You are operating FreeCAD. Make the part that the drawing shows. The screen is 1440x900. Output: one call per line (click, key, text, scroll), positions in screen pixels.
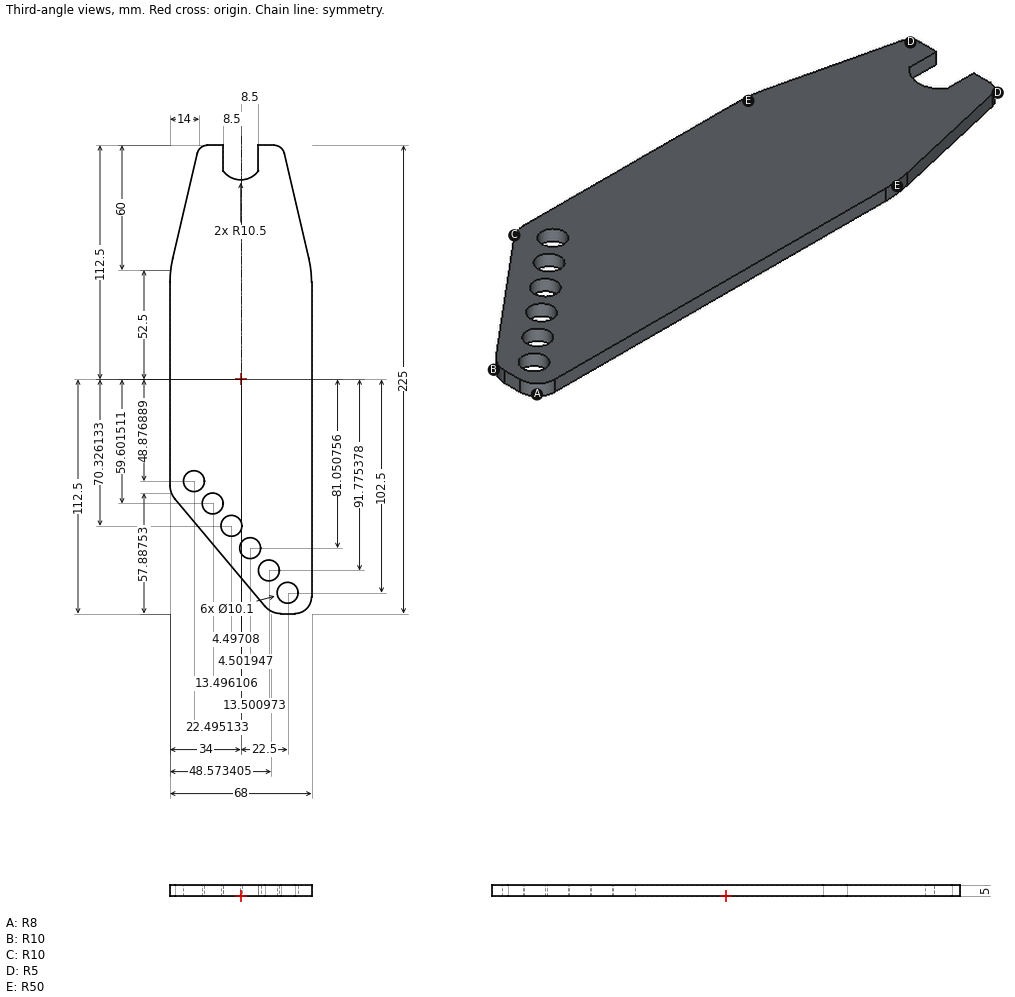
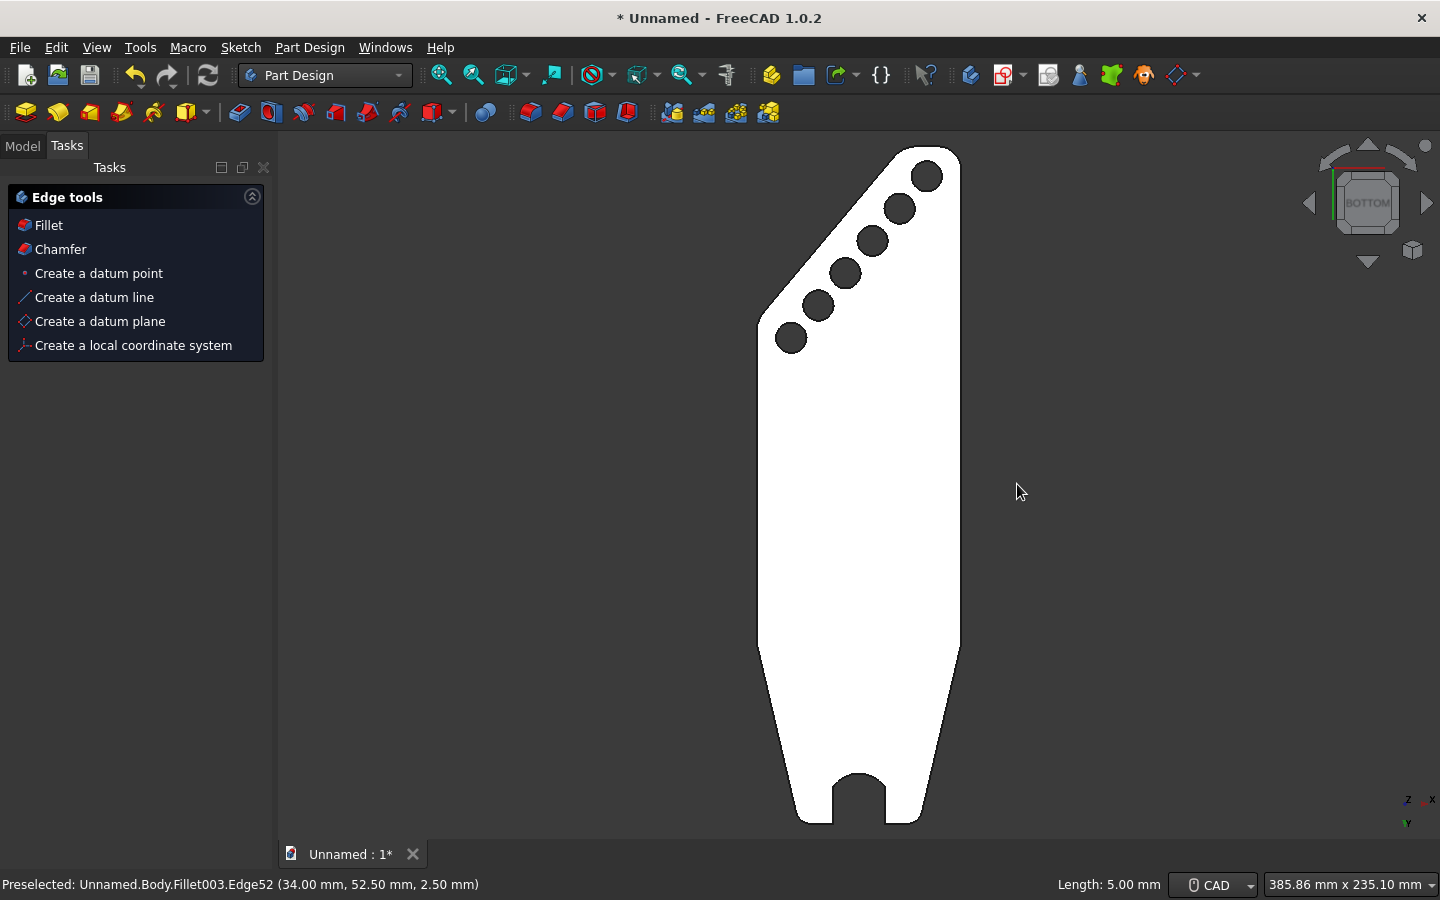
scroll(757, 642, up, 5)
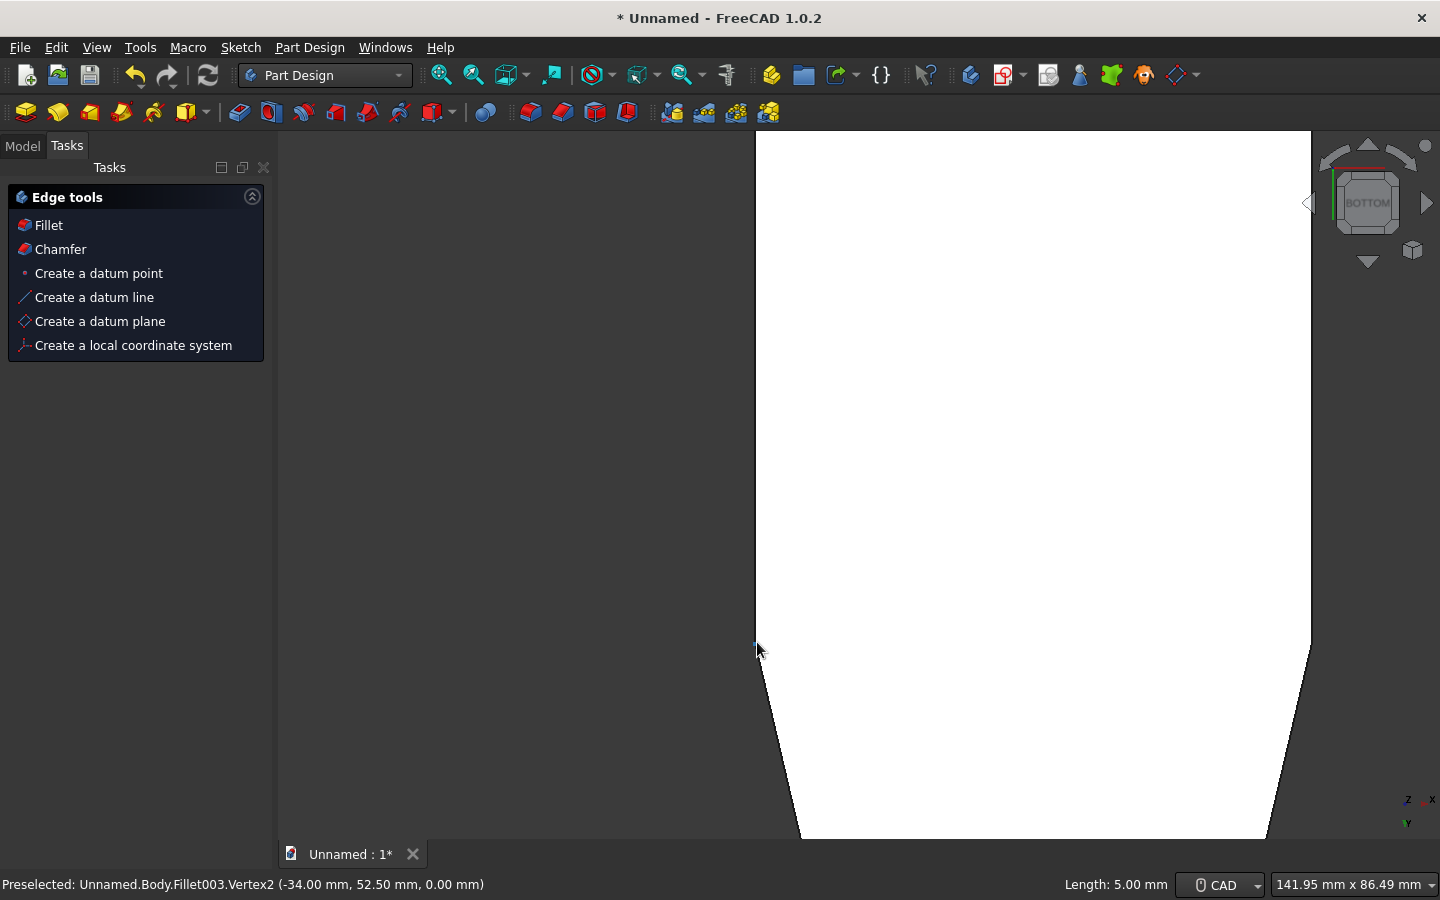
key(v)
key(f)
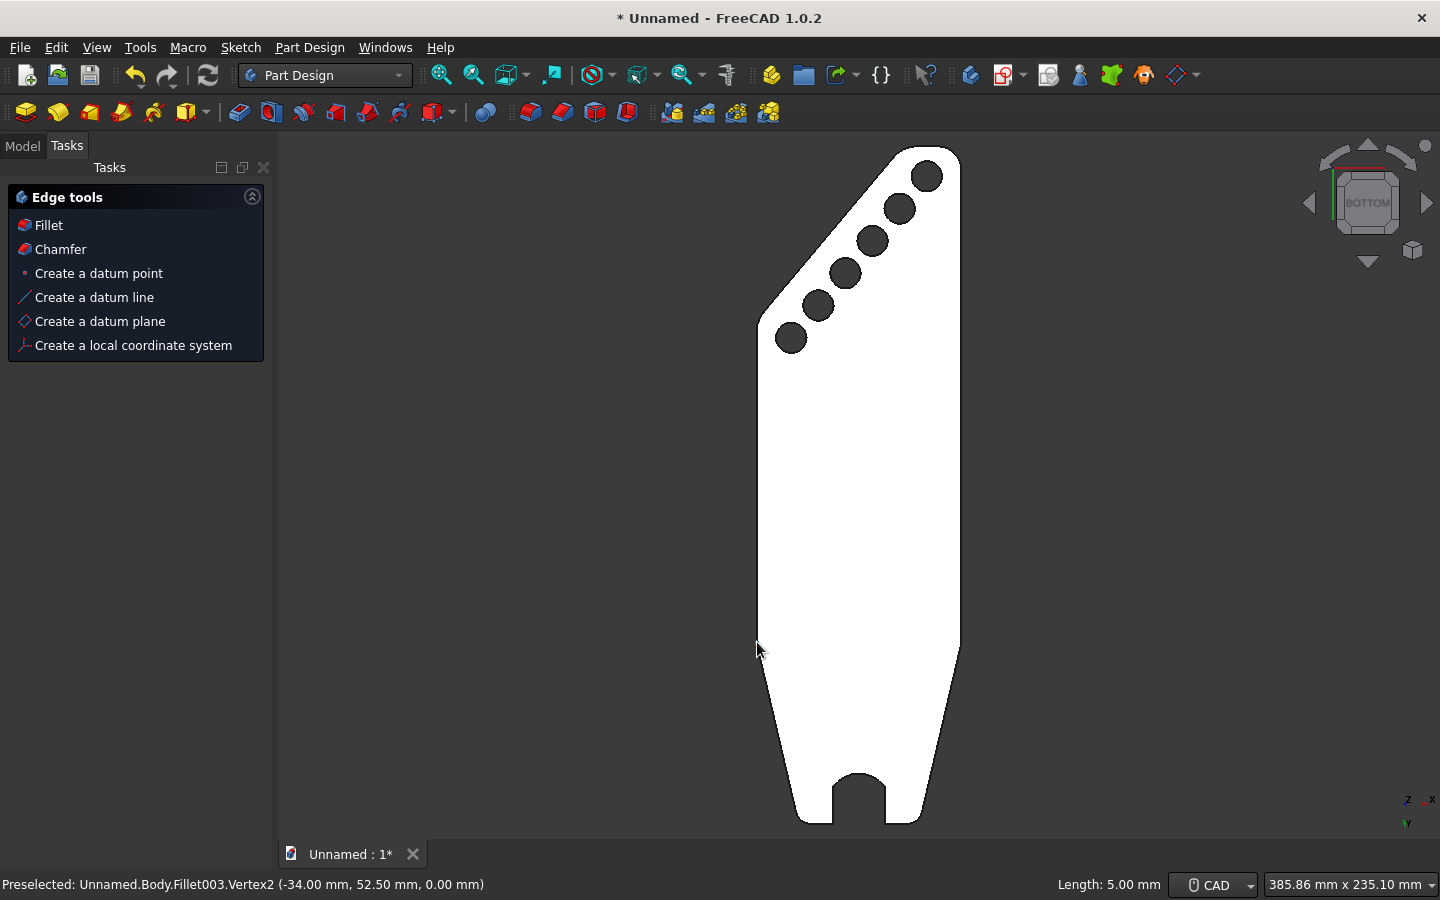
key(4)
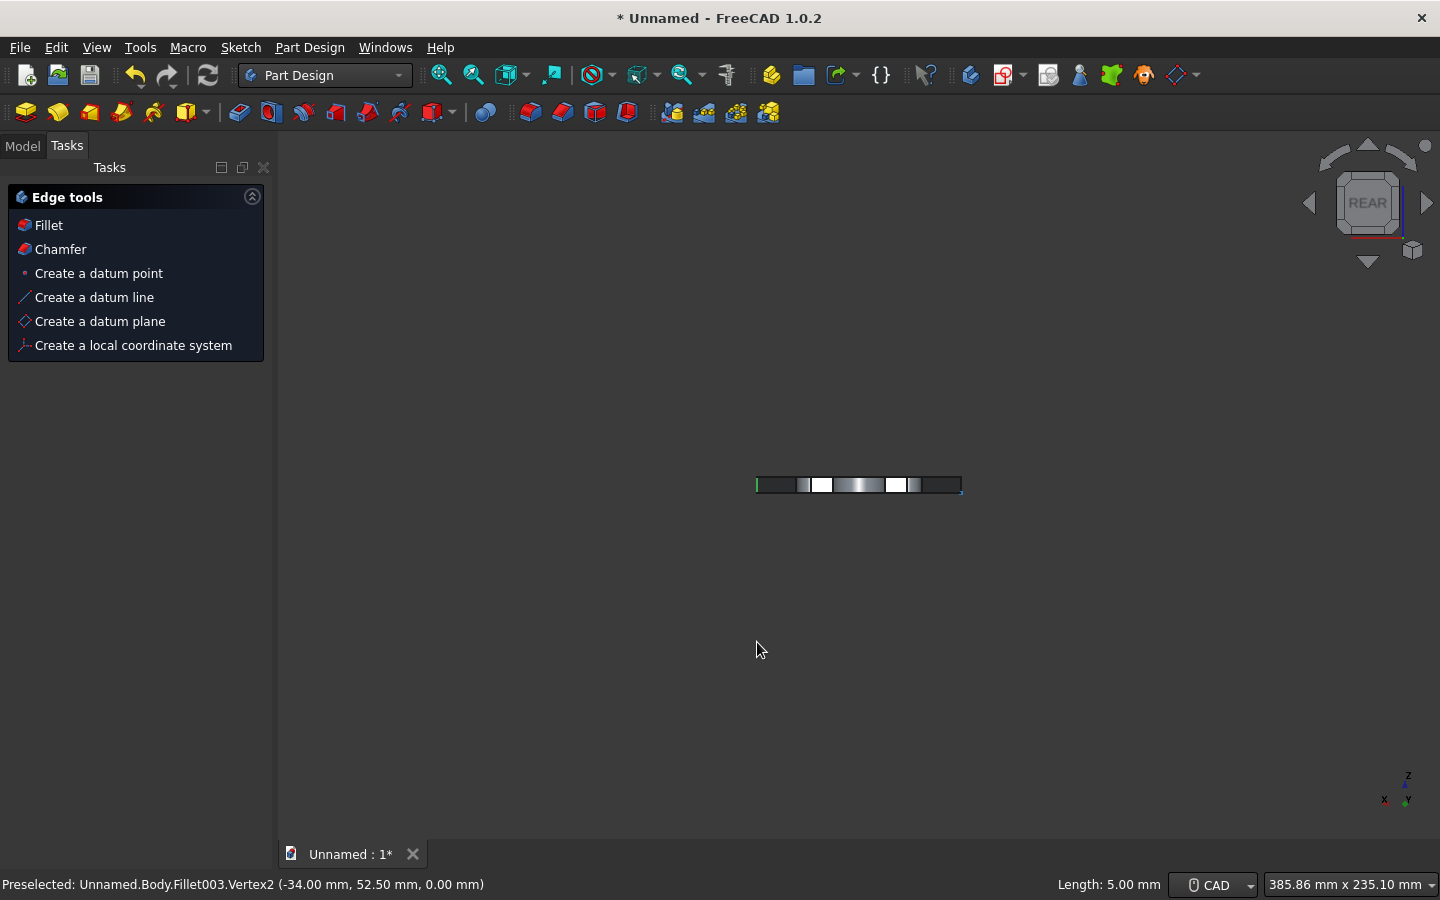
key(v)
key(f)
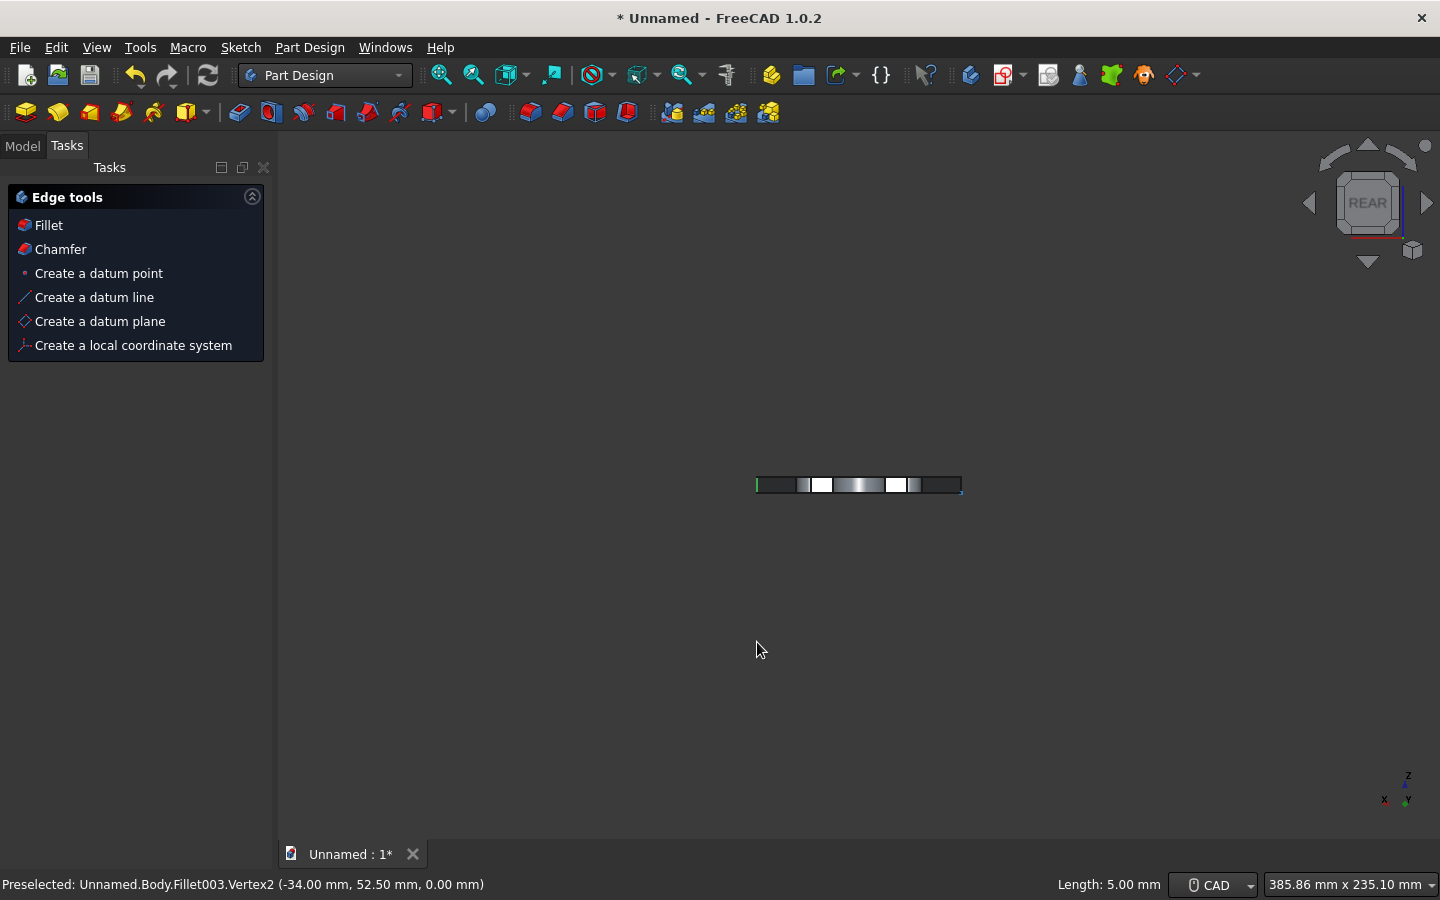
scroll(961, 484, up, 5)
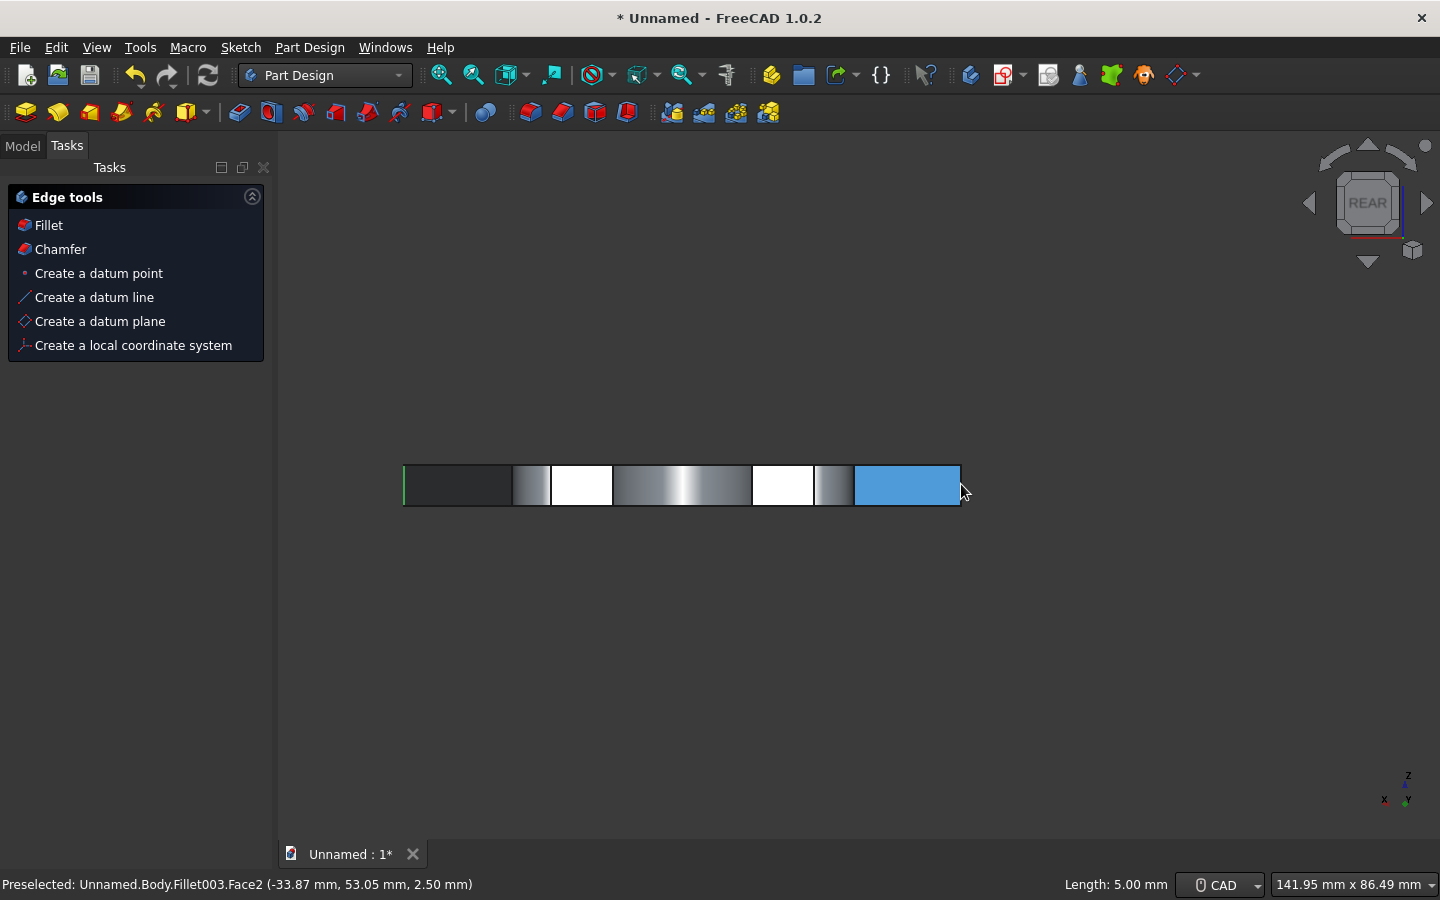
click(442, 76)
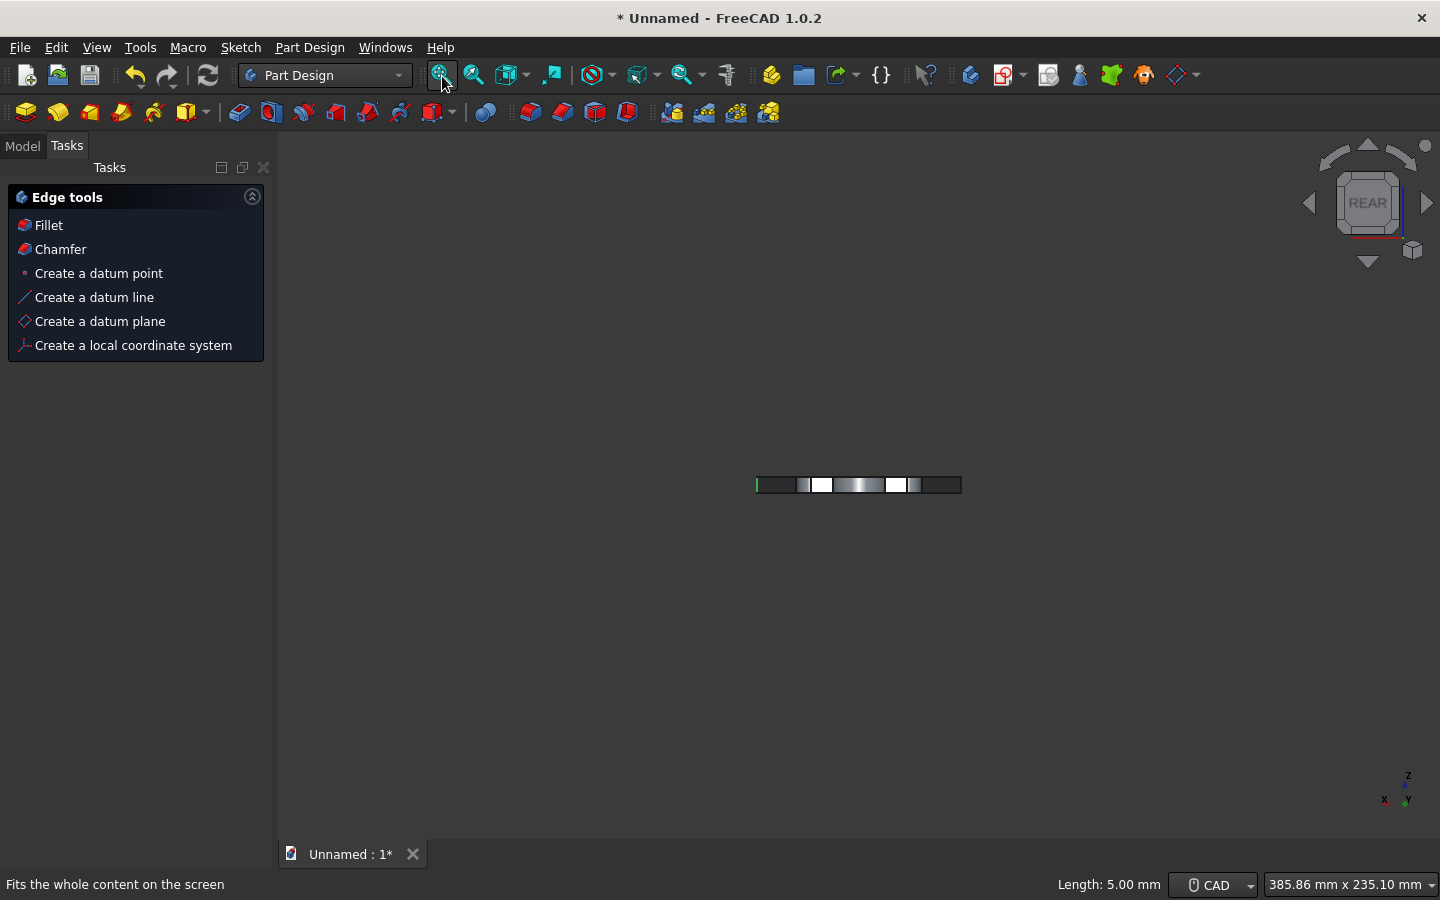
key(6)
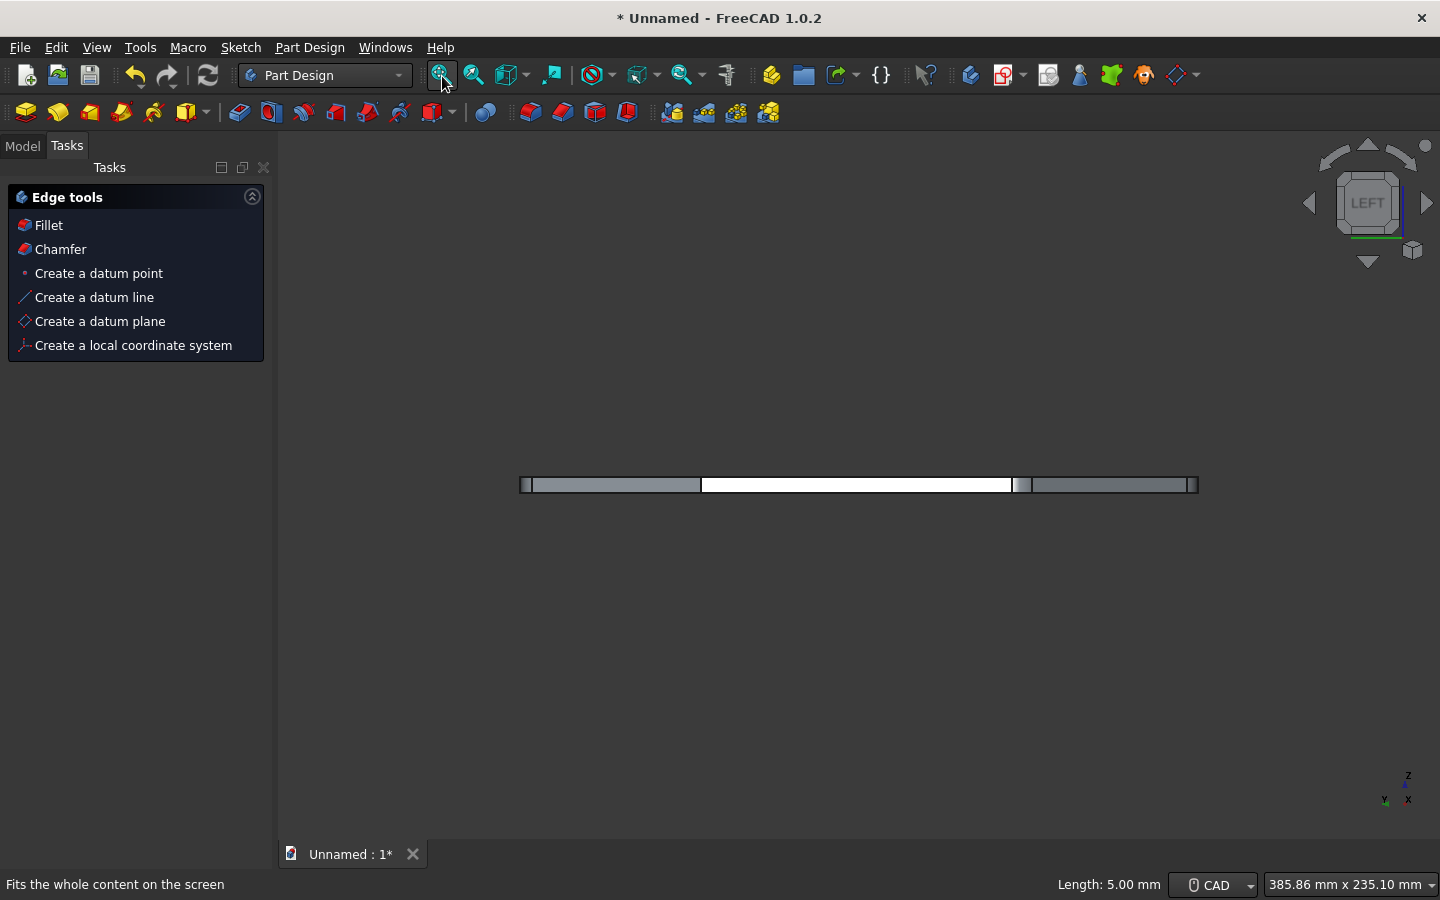
click(701, 484, ctrl)